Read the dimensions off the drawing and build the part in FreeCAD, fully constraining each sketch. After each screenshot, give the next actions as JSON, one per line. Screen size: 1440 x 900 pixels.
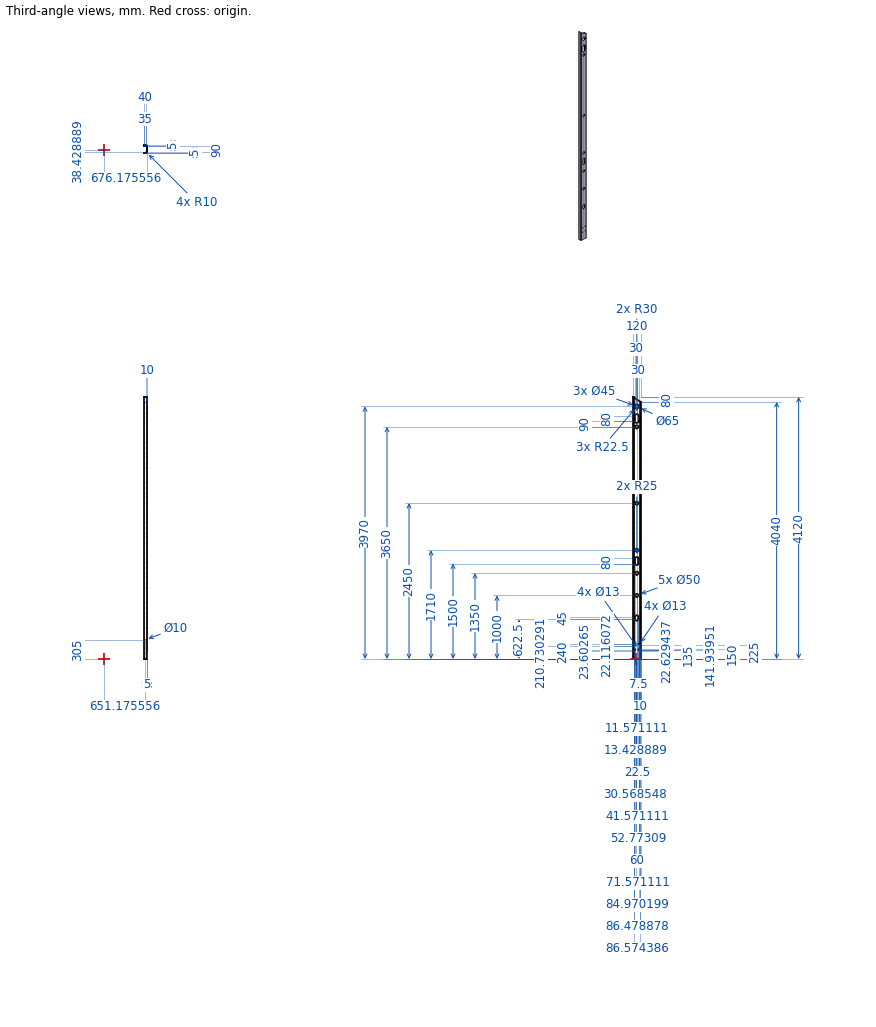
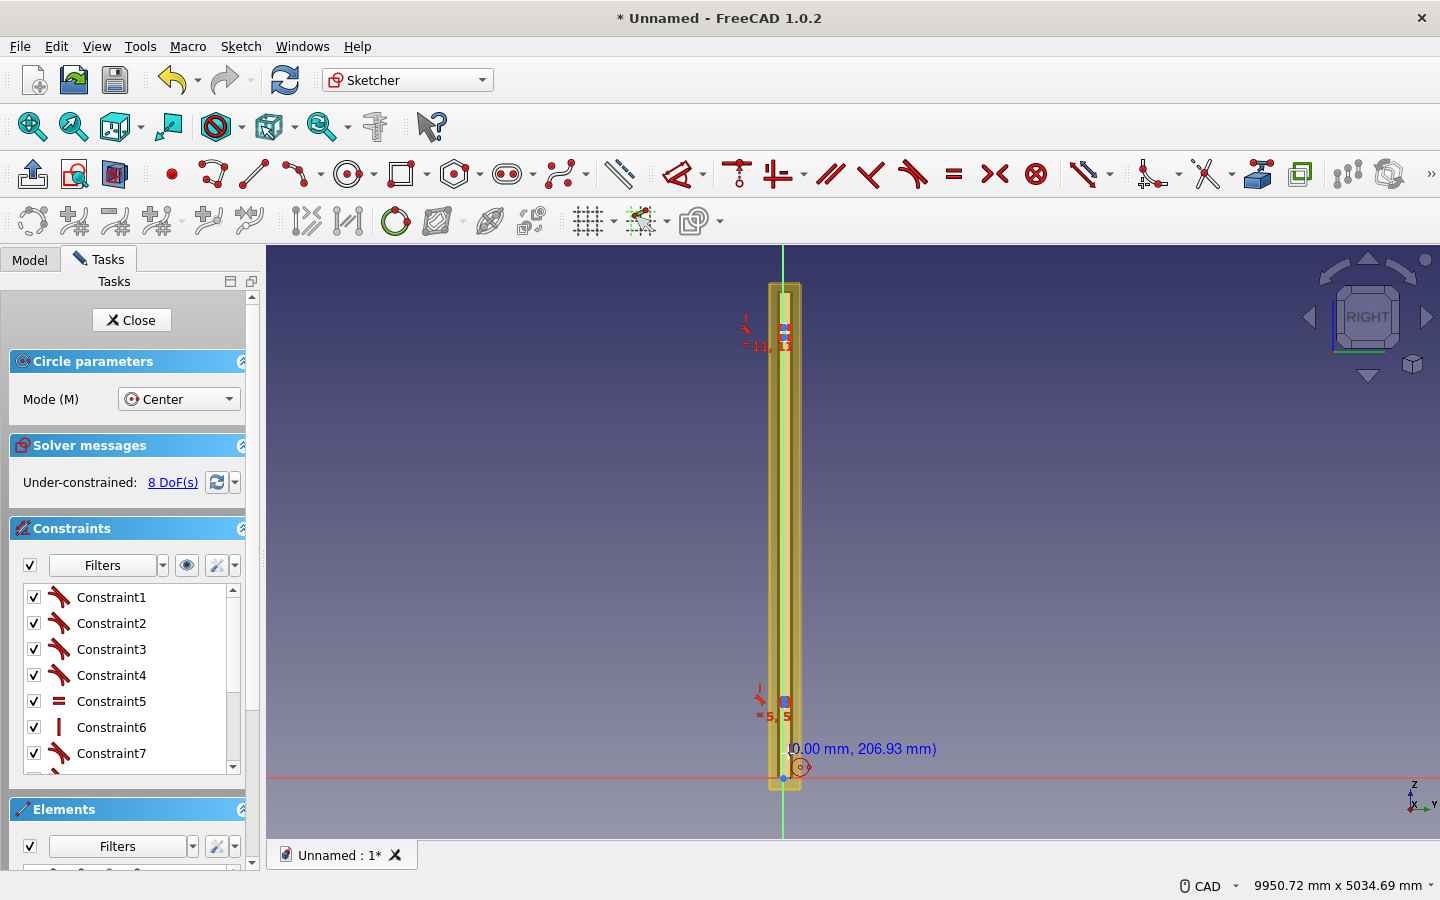
{"action": "scroll", "coordinate": [788, 752], "scroll_direction": "up", "scroll_amount": 6}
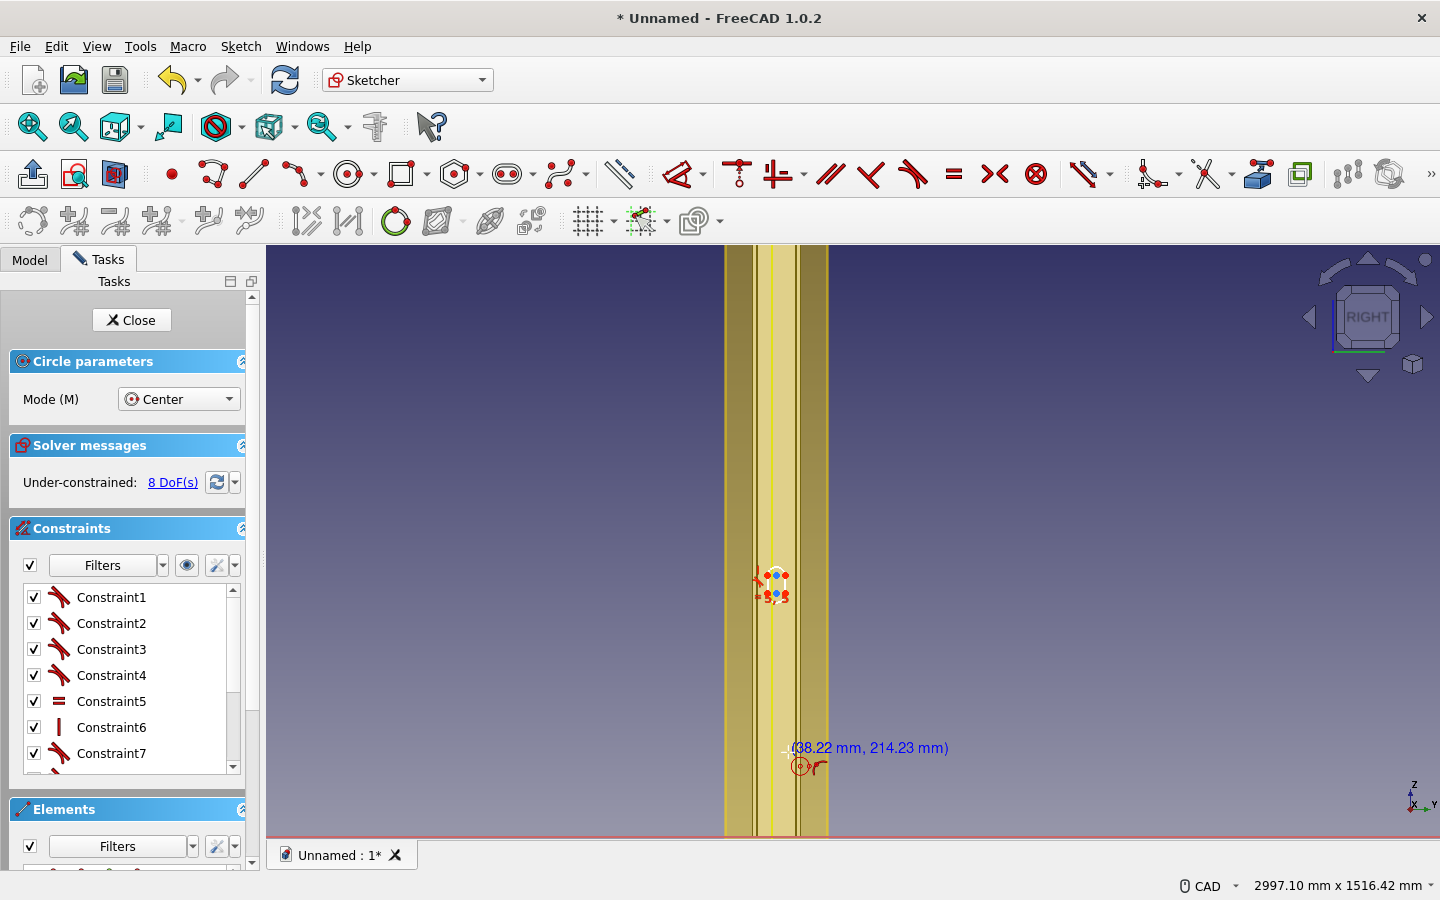
{"action": "left_click", "coordinate": [788, 749]}
{"action": "mouse_move", "coordinate": [790, 747]}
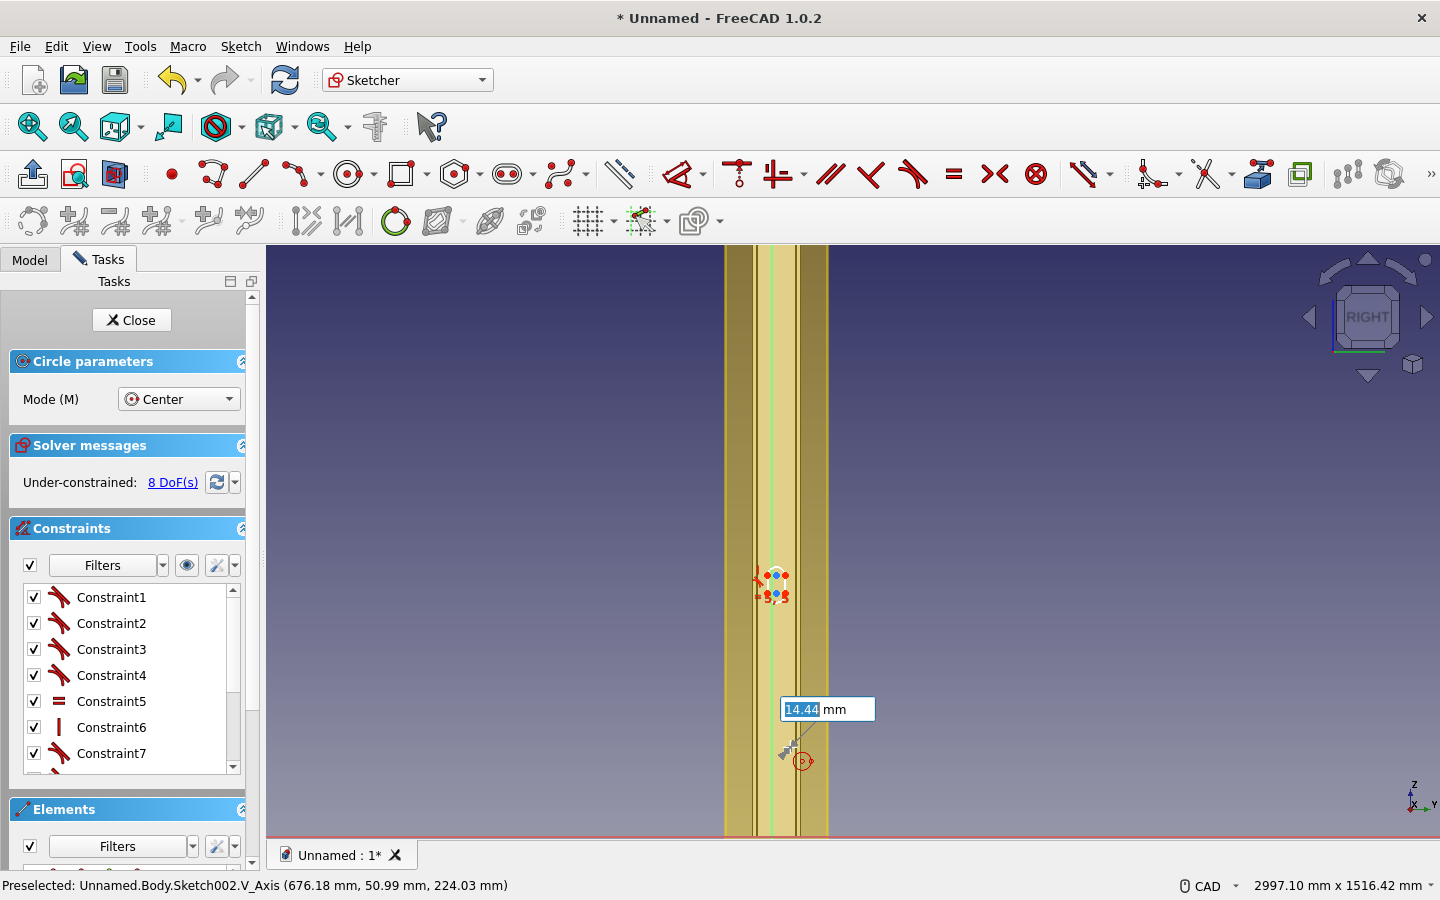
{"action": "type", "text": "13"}
{"action": "key", "text": "Return"}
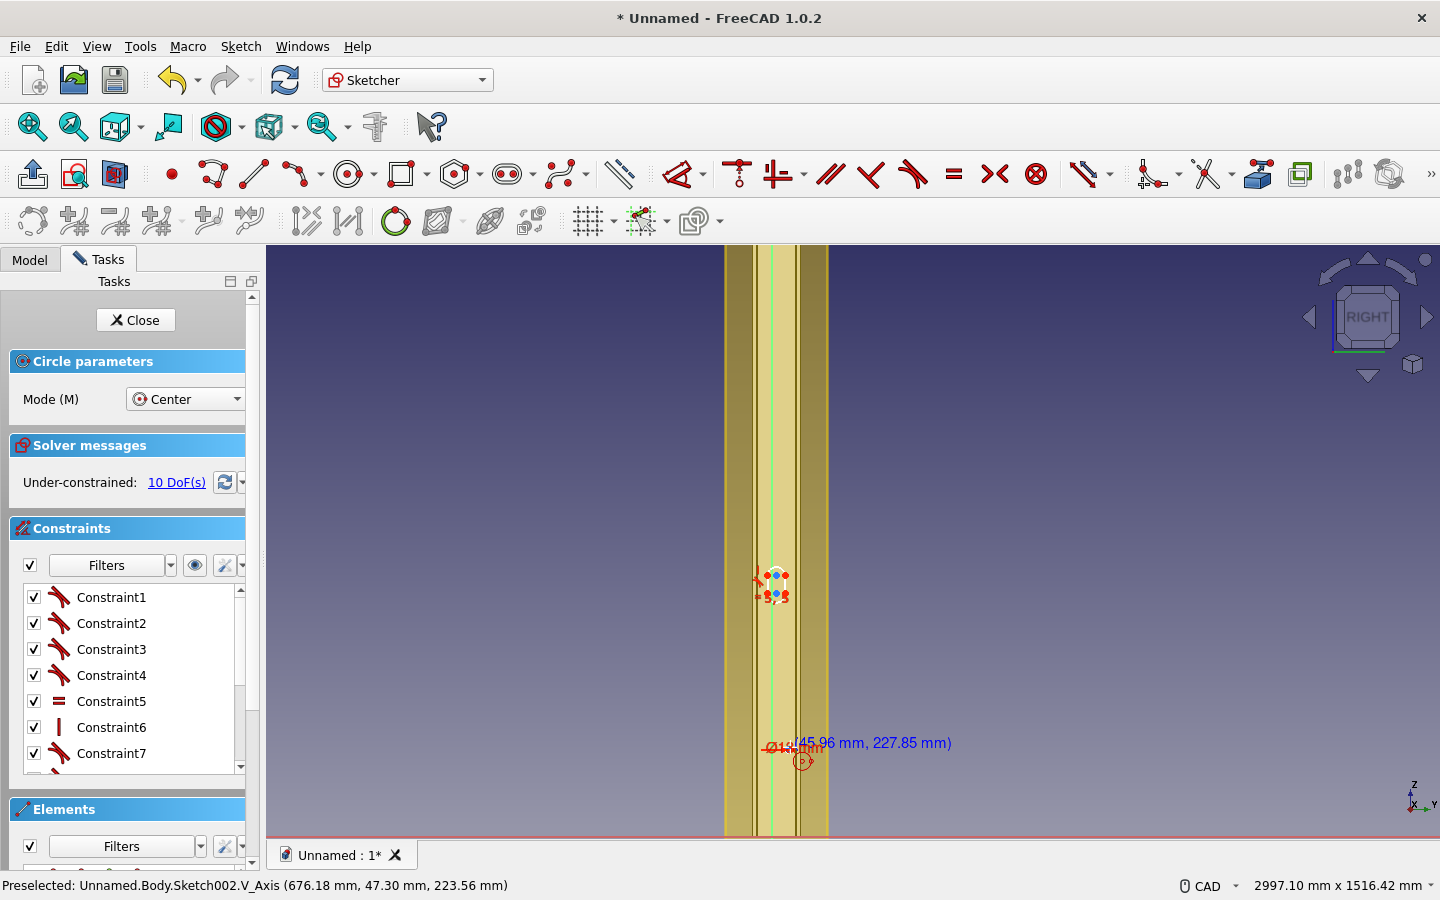
{"action": "scroll", "coordinate": [788, 784], "scroll_direction": "up", "scroll_amount": 11}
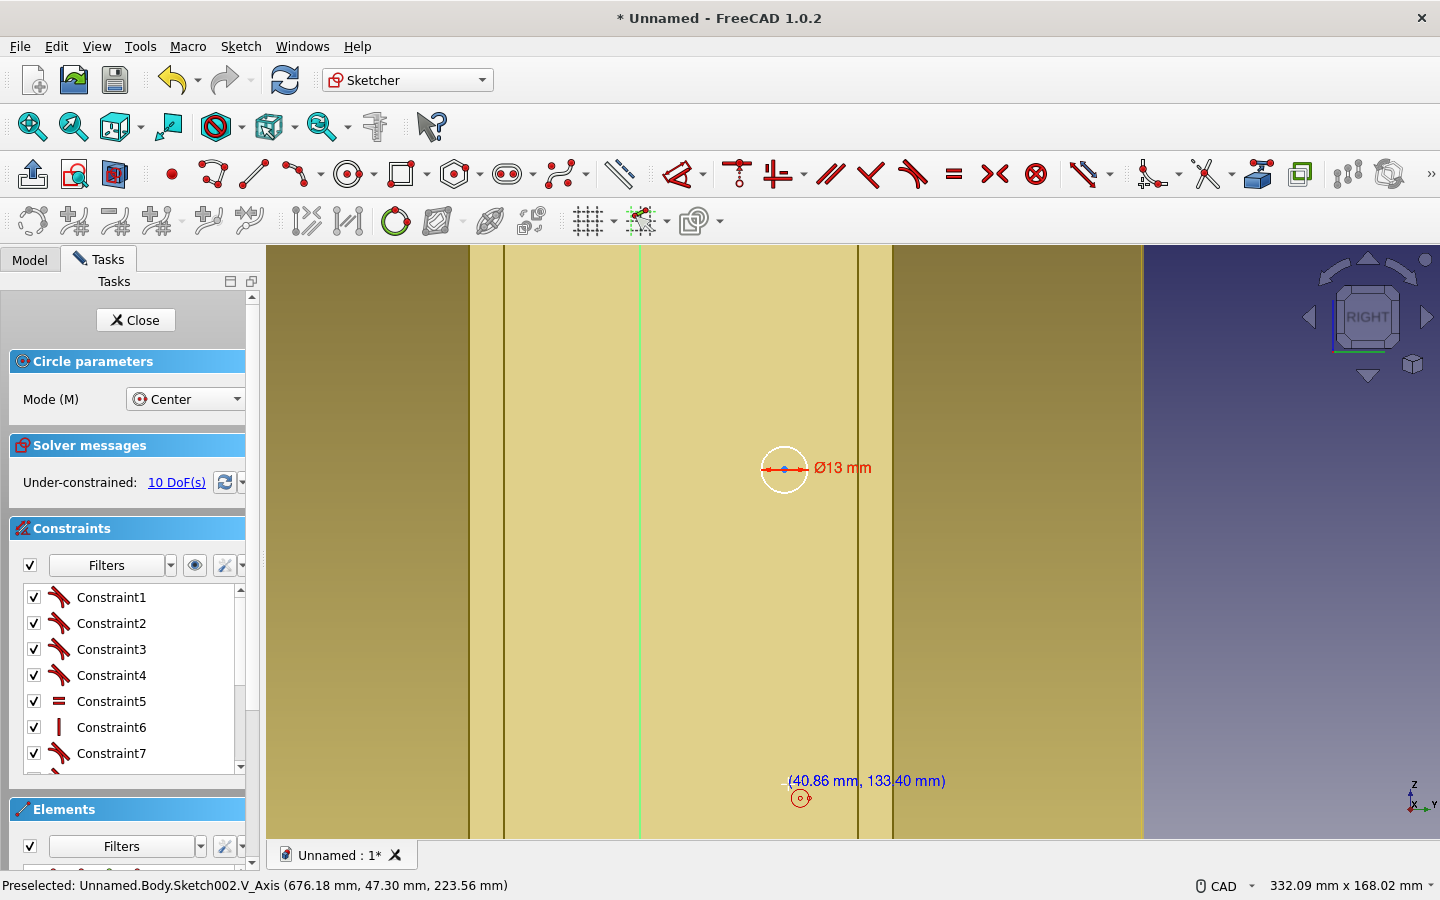
{"action": "scroll", "coordinate": [788, 761], "scroll_direction": "down", "scroll_amount": 17}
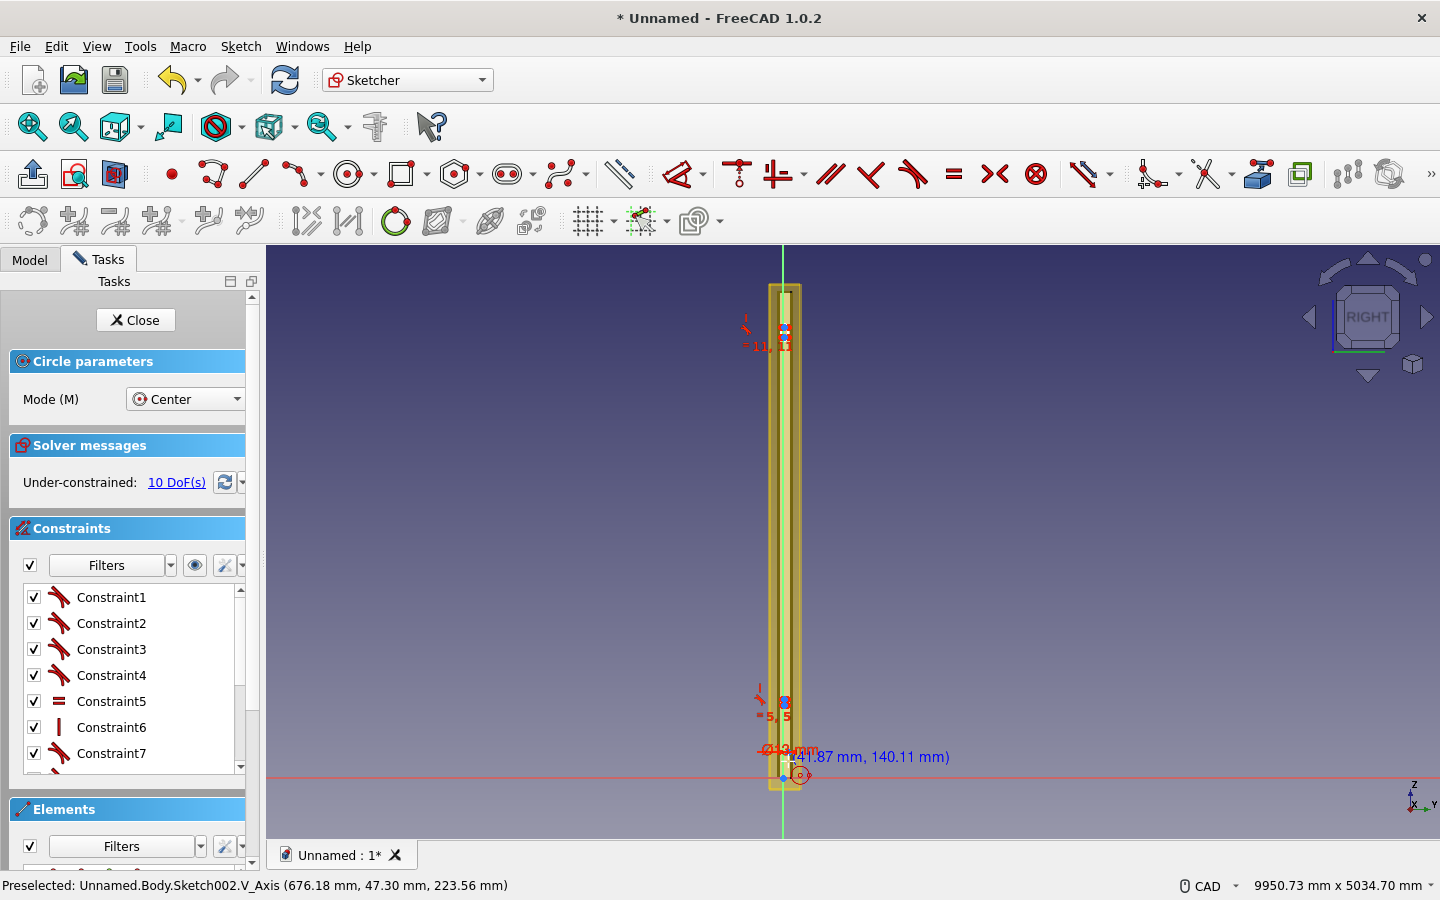
{"action": "scroll", "coordinate": [788, 762], "scroll_direction": "up", "scroll_amount": 6}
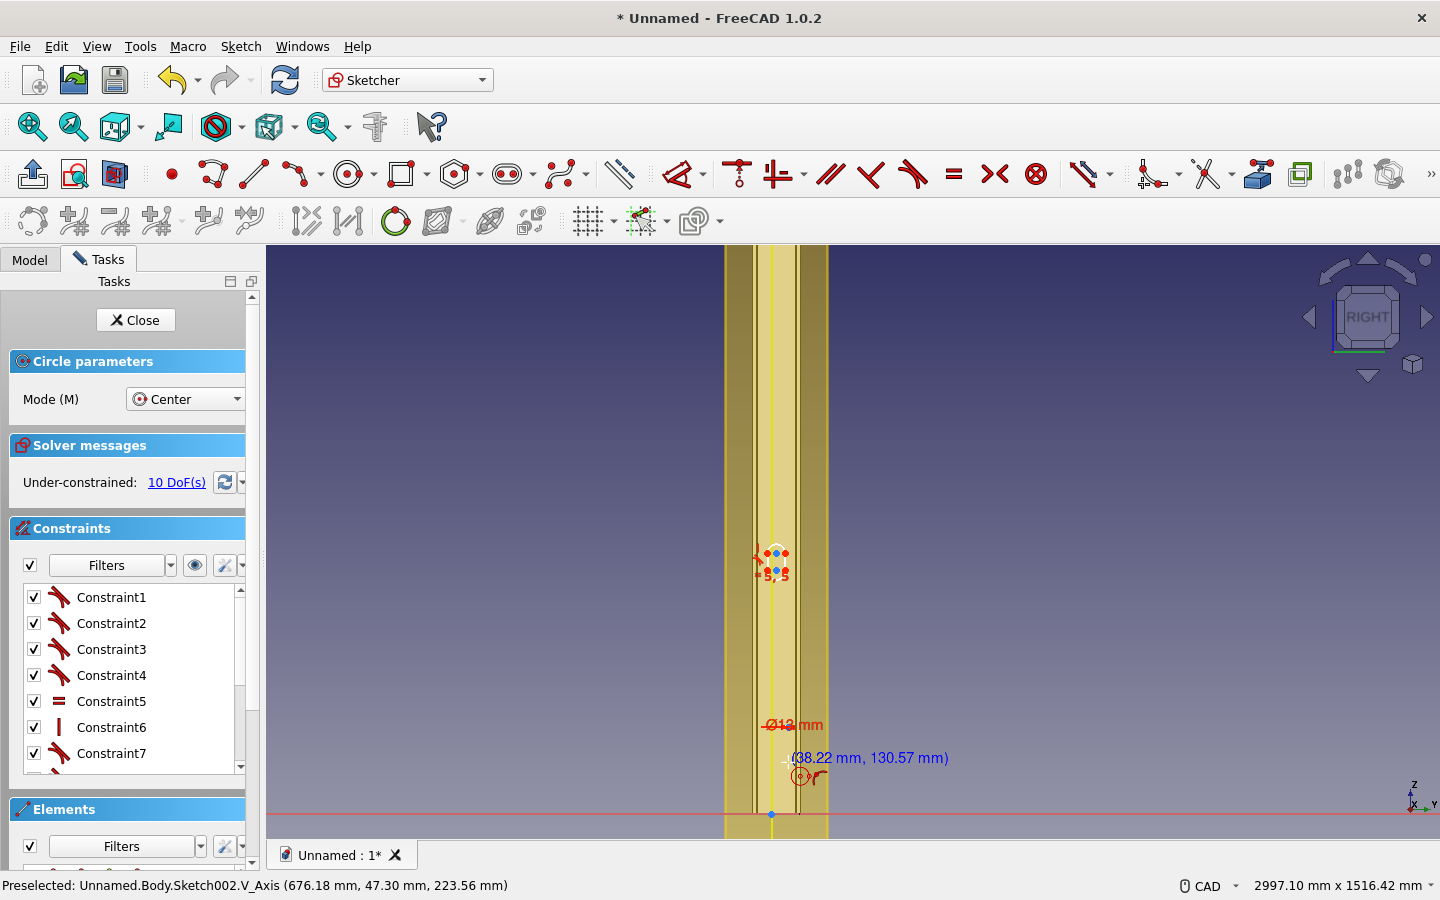
{"action": "left_click", "coordinate": [788, 762]}
{"action": "mouse_move", "coordinate": [790, 760]}